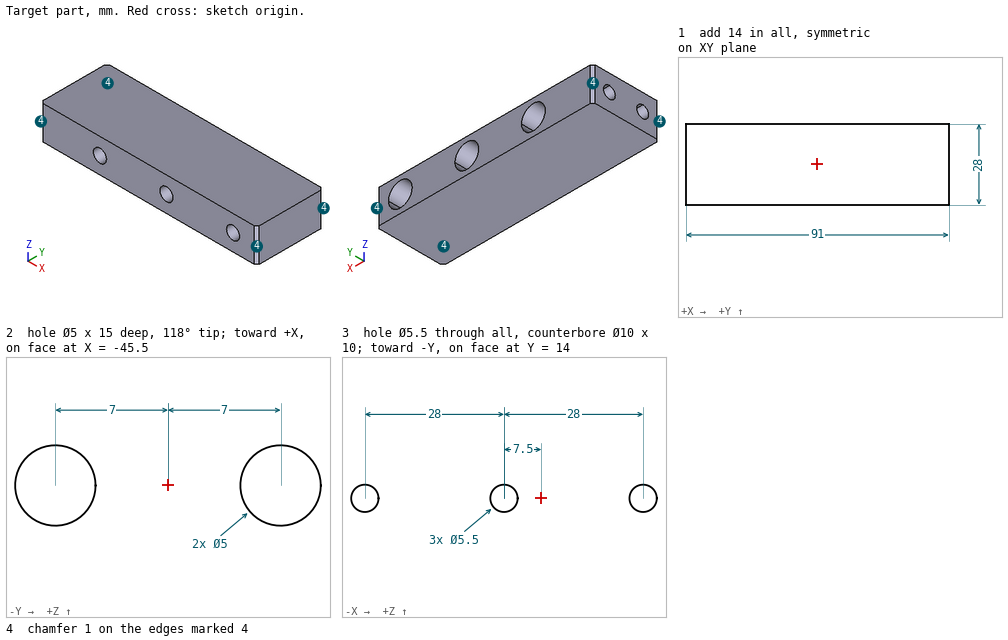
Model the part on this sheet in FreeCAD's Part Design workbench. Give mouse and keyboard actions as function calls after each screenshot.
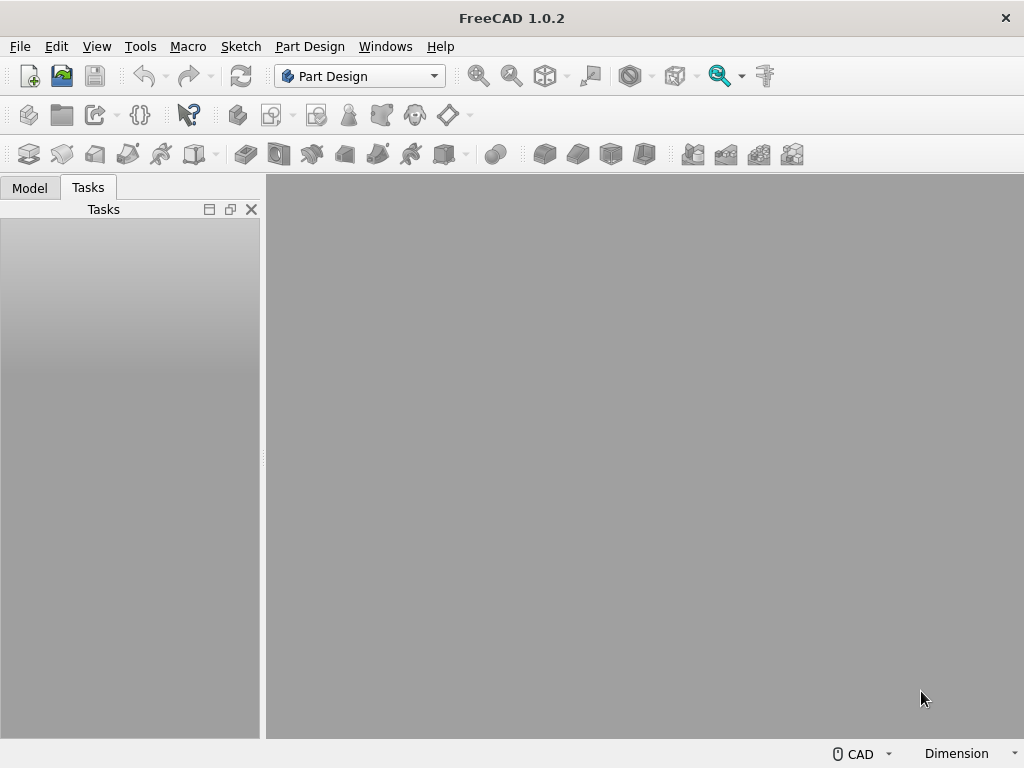
click(29, 76)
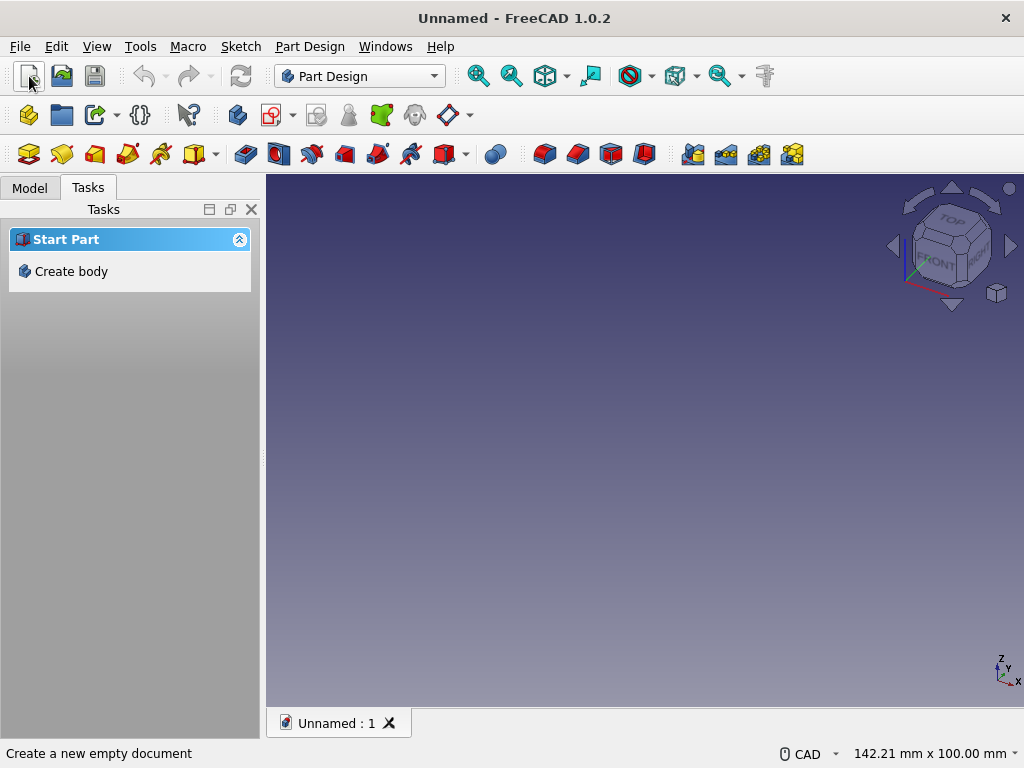
click(270, 116)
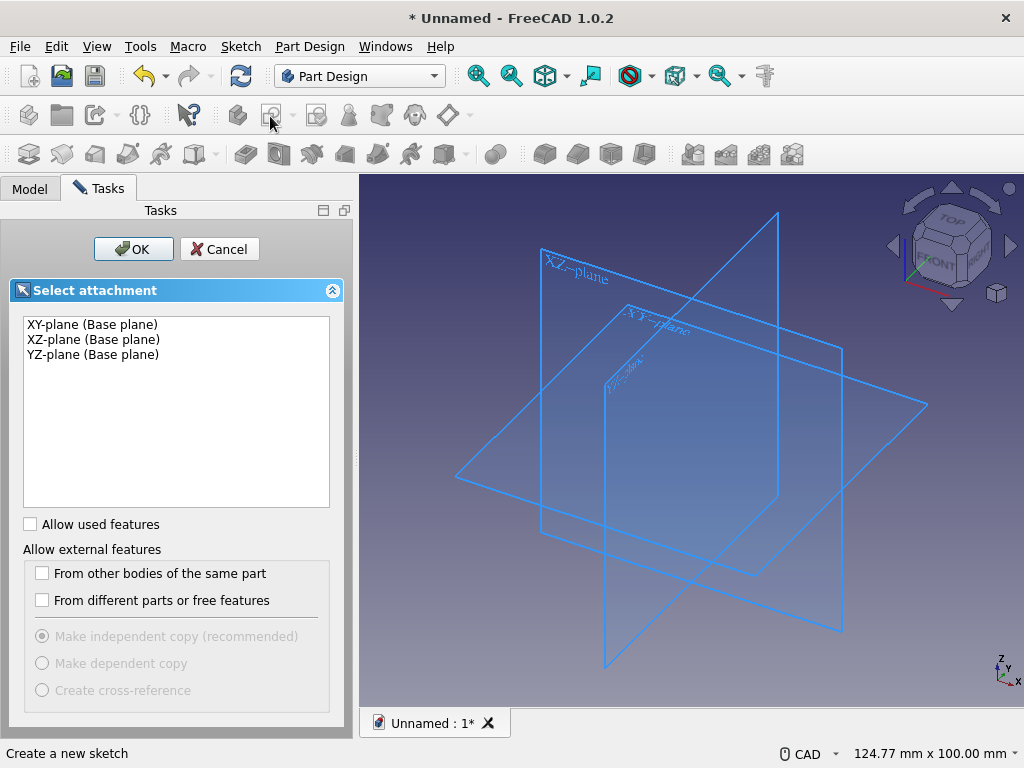
click(84, 324)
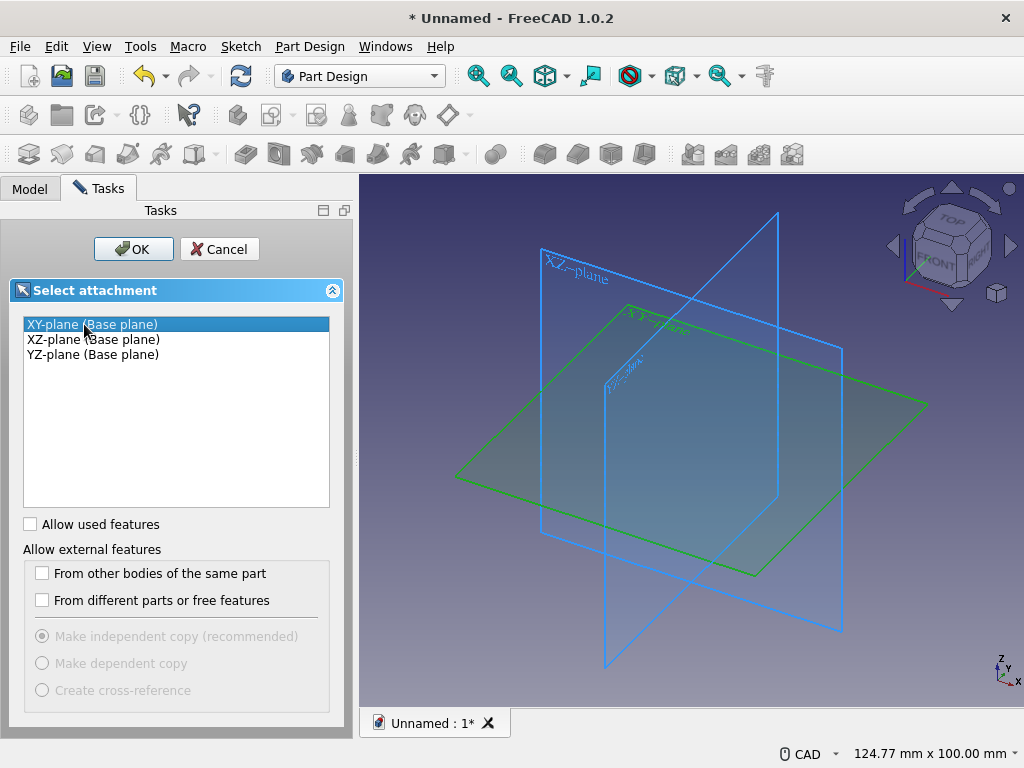
click(134, 249)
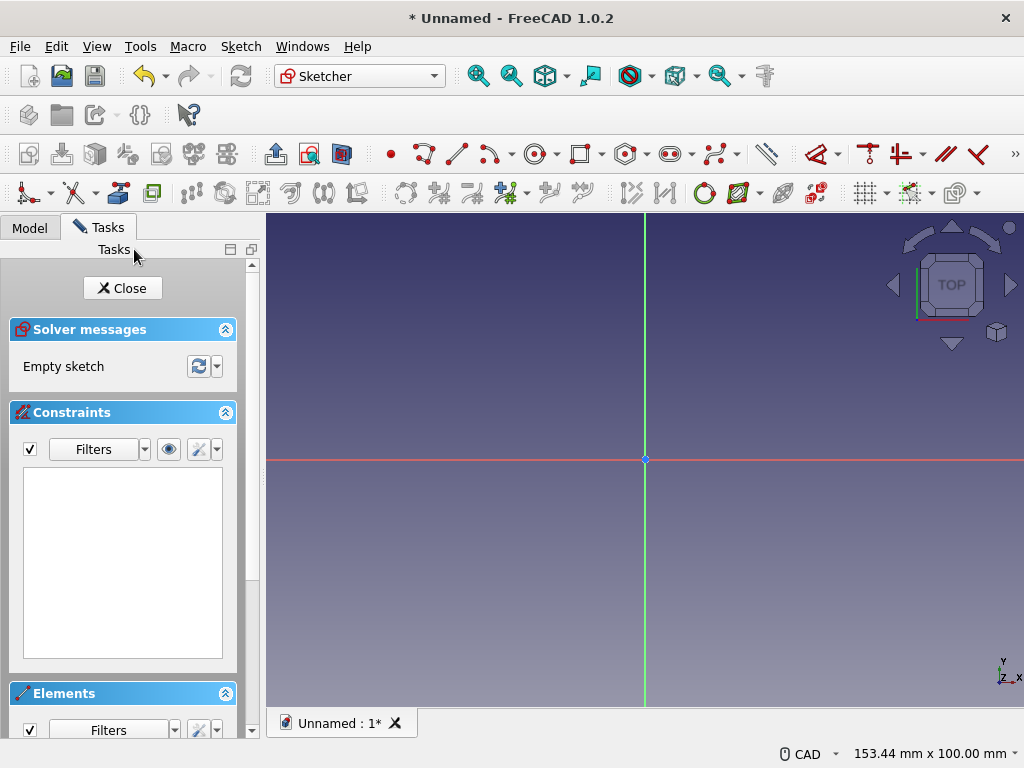
scroll(294, 460, down, 1)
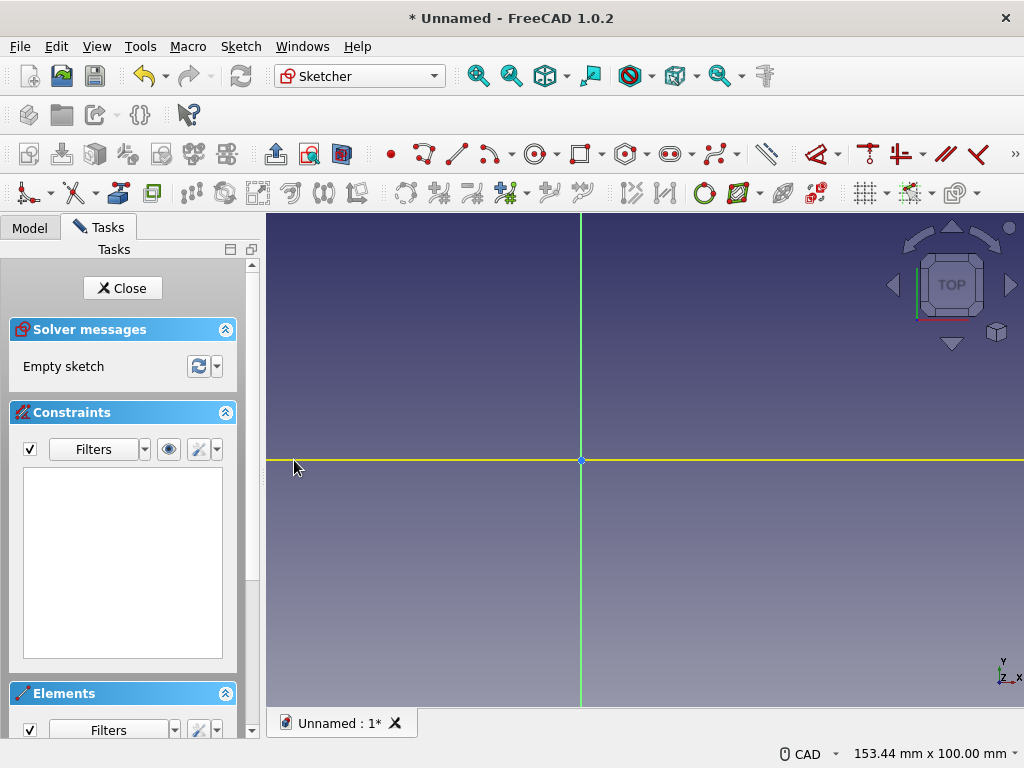
key(g)
key(v)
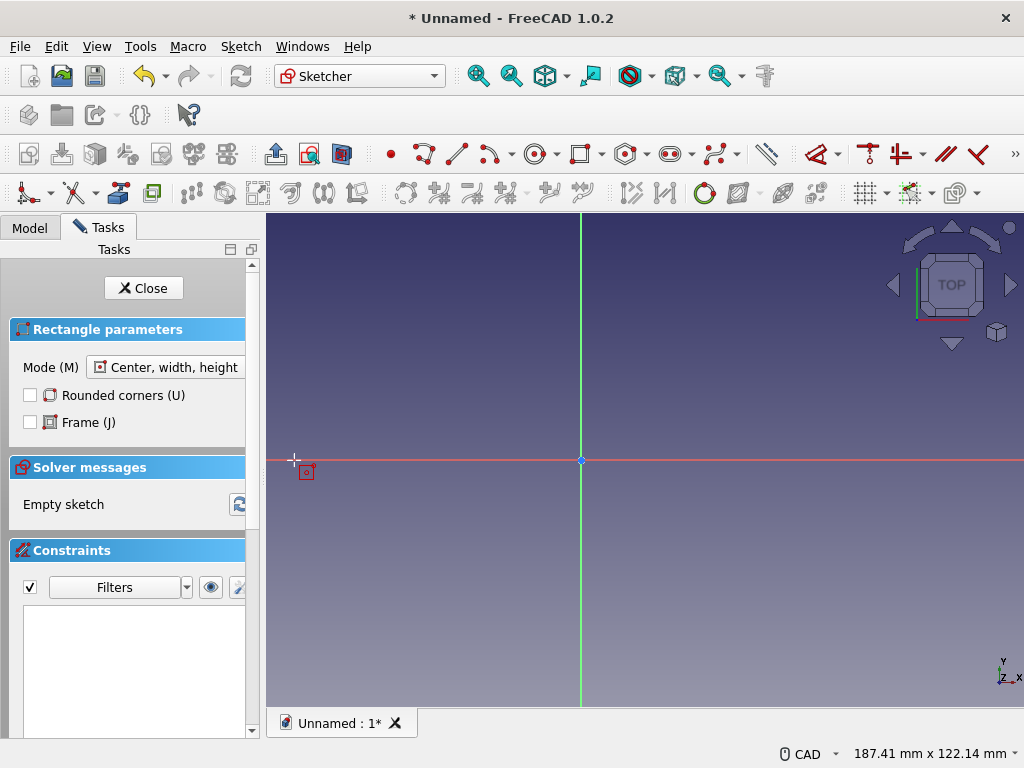
click(581, 460)
move(765, 403)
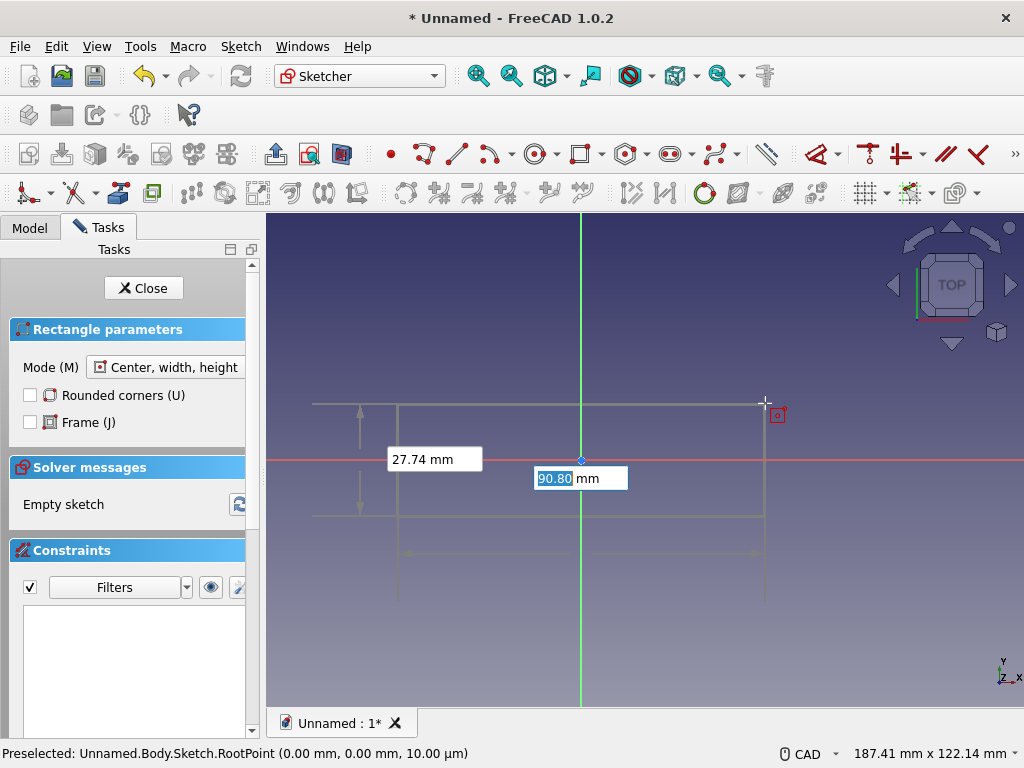
text(91)
key(Tab)
text(28)
key(Return)
key(Escape)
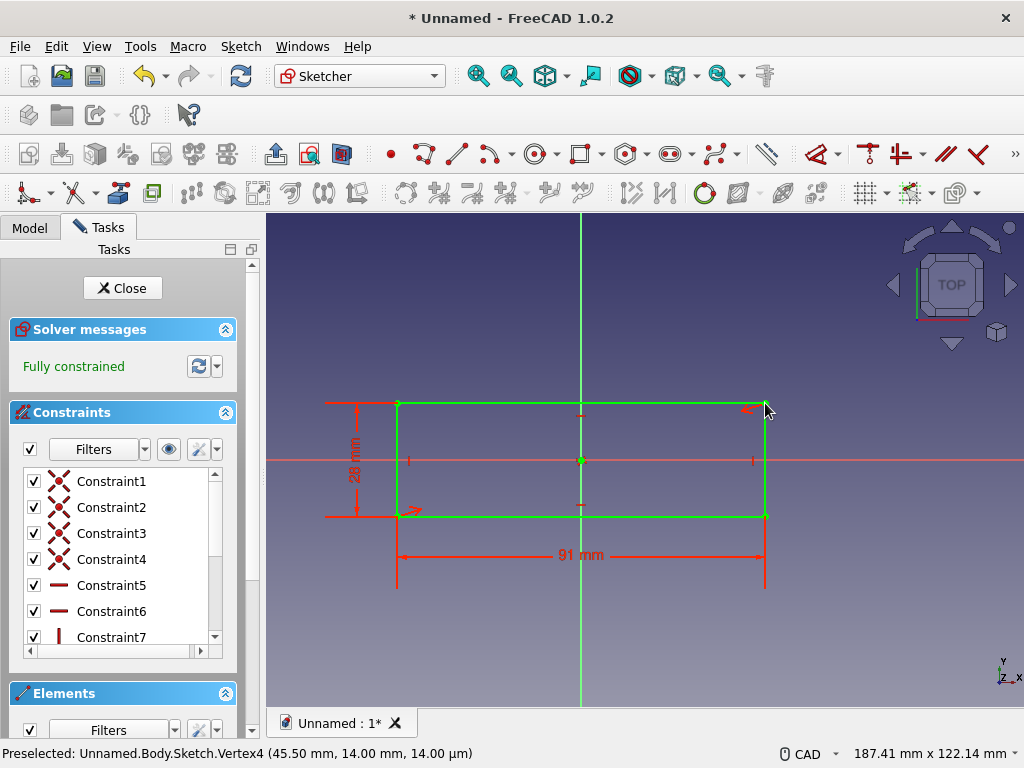
click(123, 288)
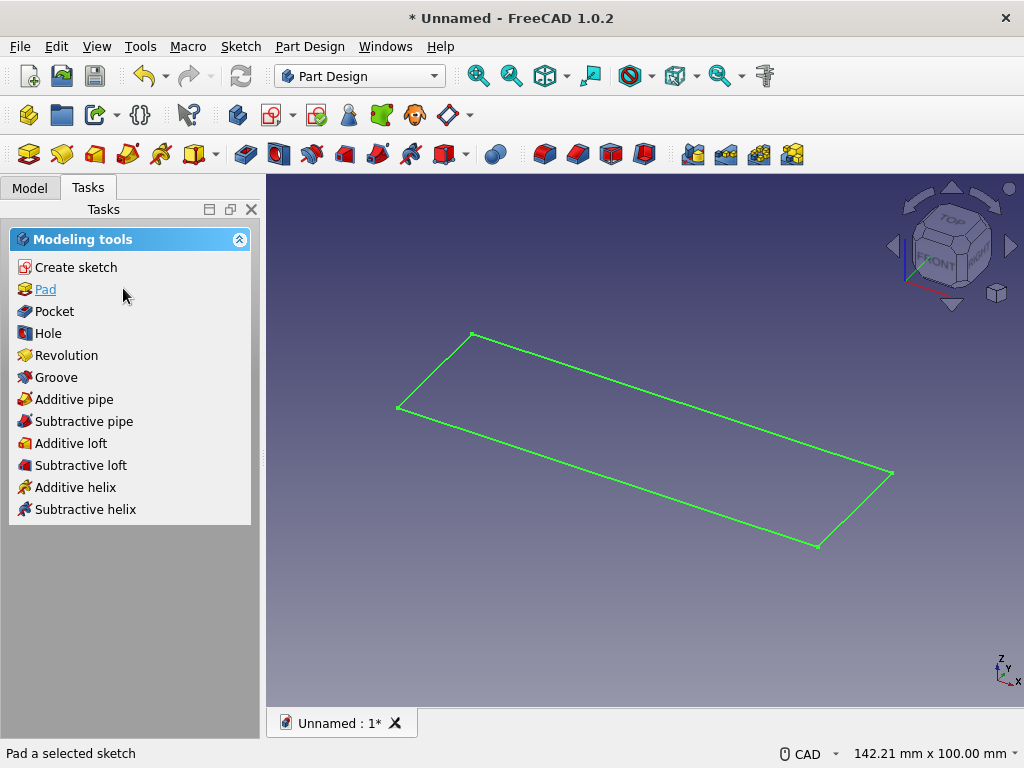
click(29, 154)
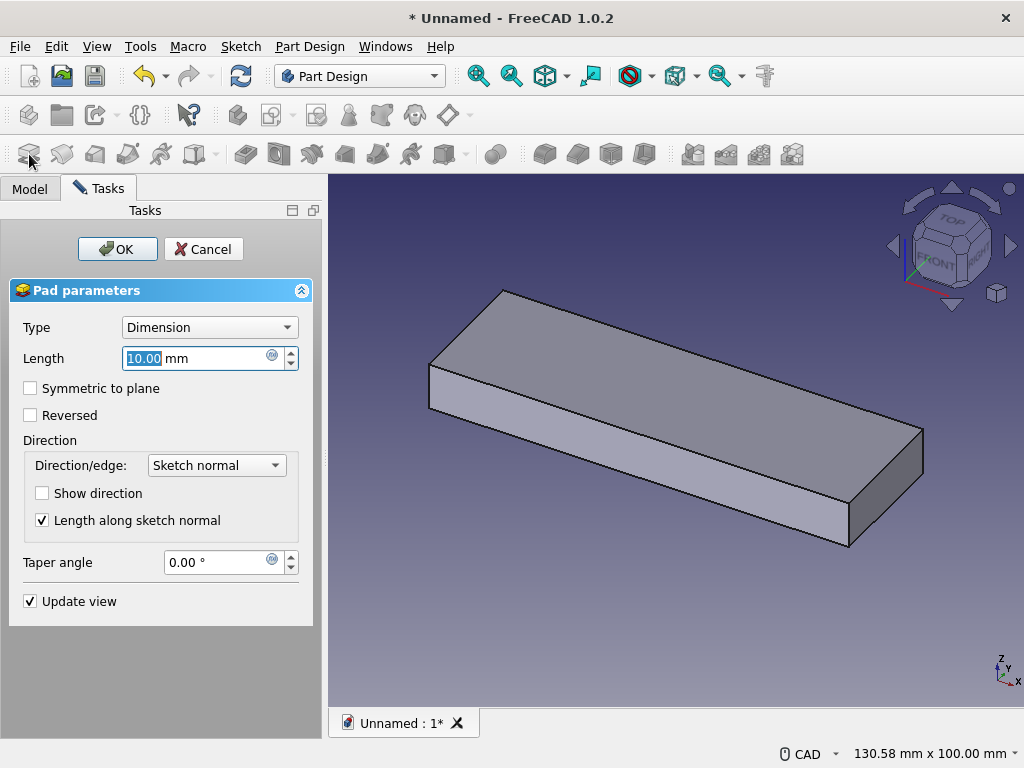
text(14)
key(Tab)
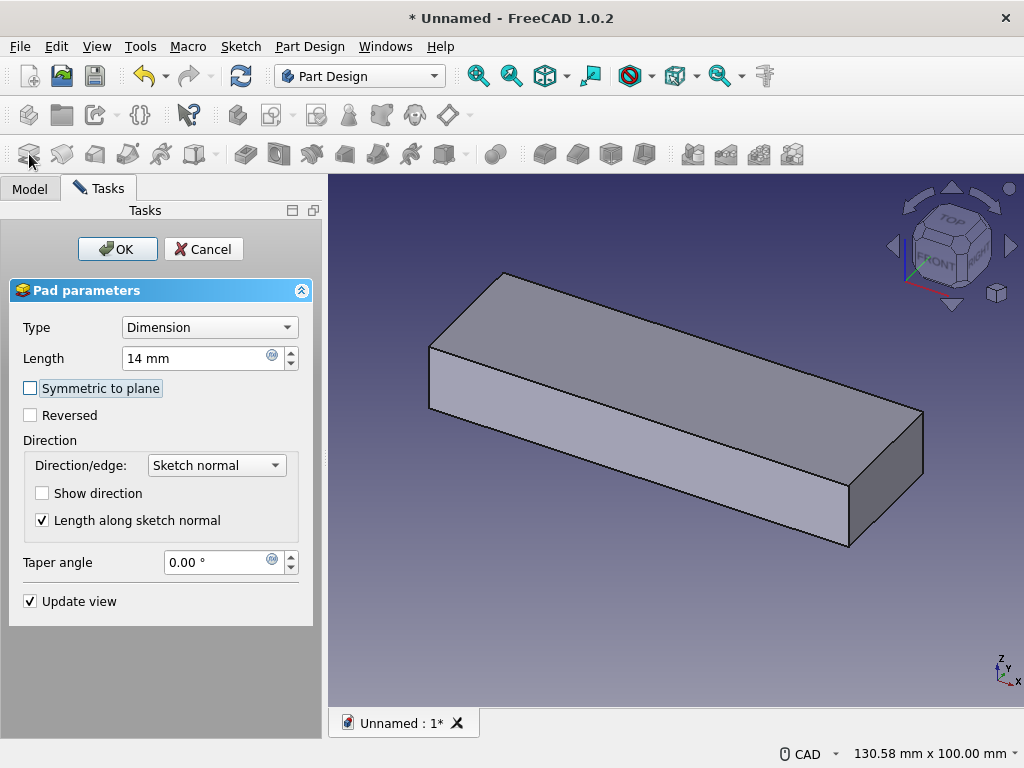
click(31, 388)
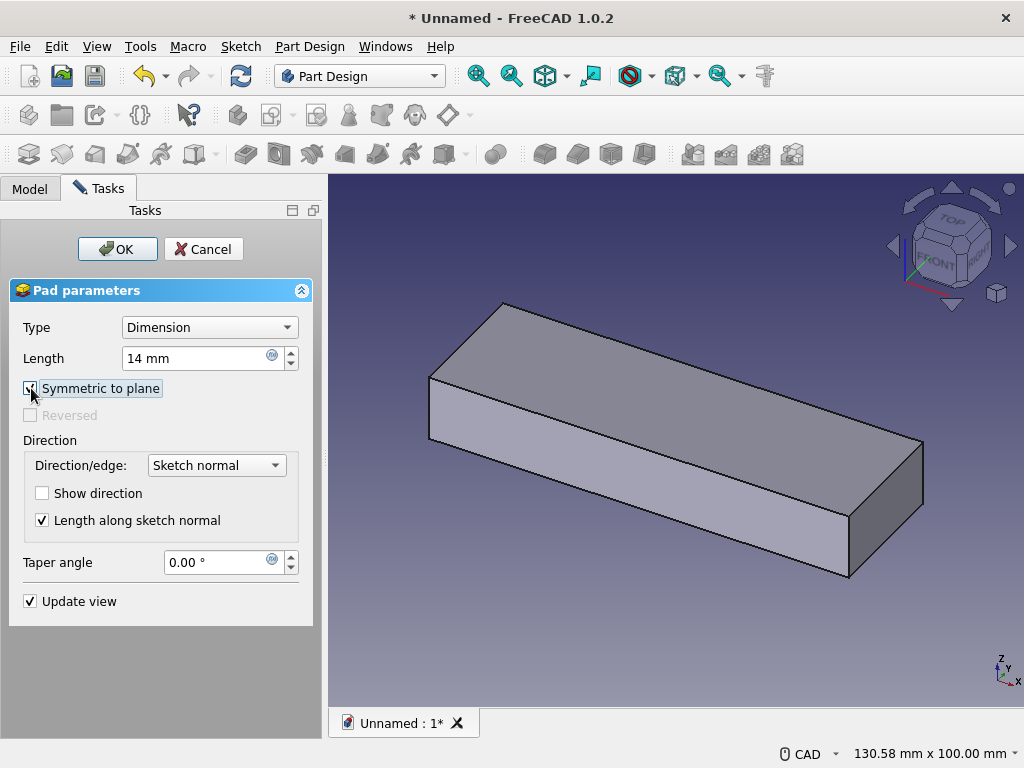
click(118, 249)